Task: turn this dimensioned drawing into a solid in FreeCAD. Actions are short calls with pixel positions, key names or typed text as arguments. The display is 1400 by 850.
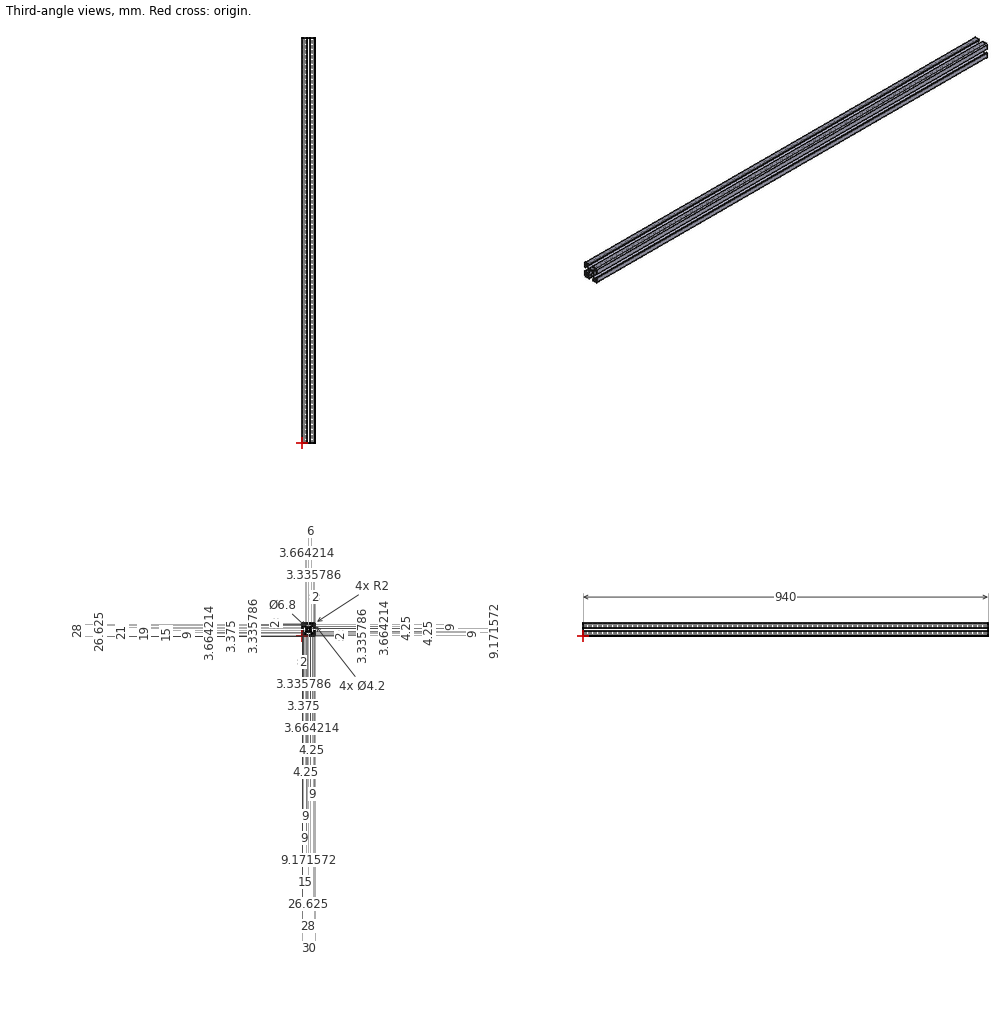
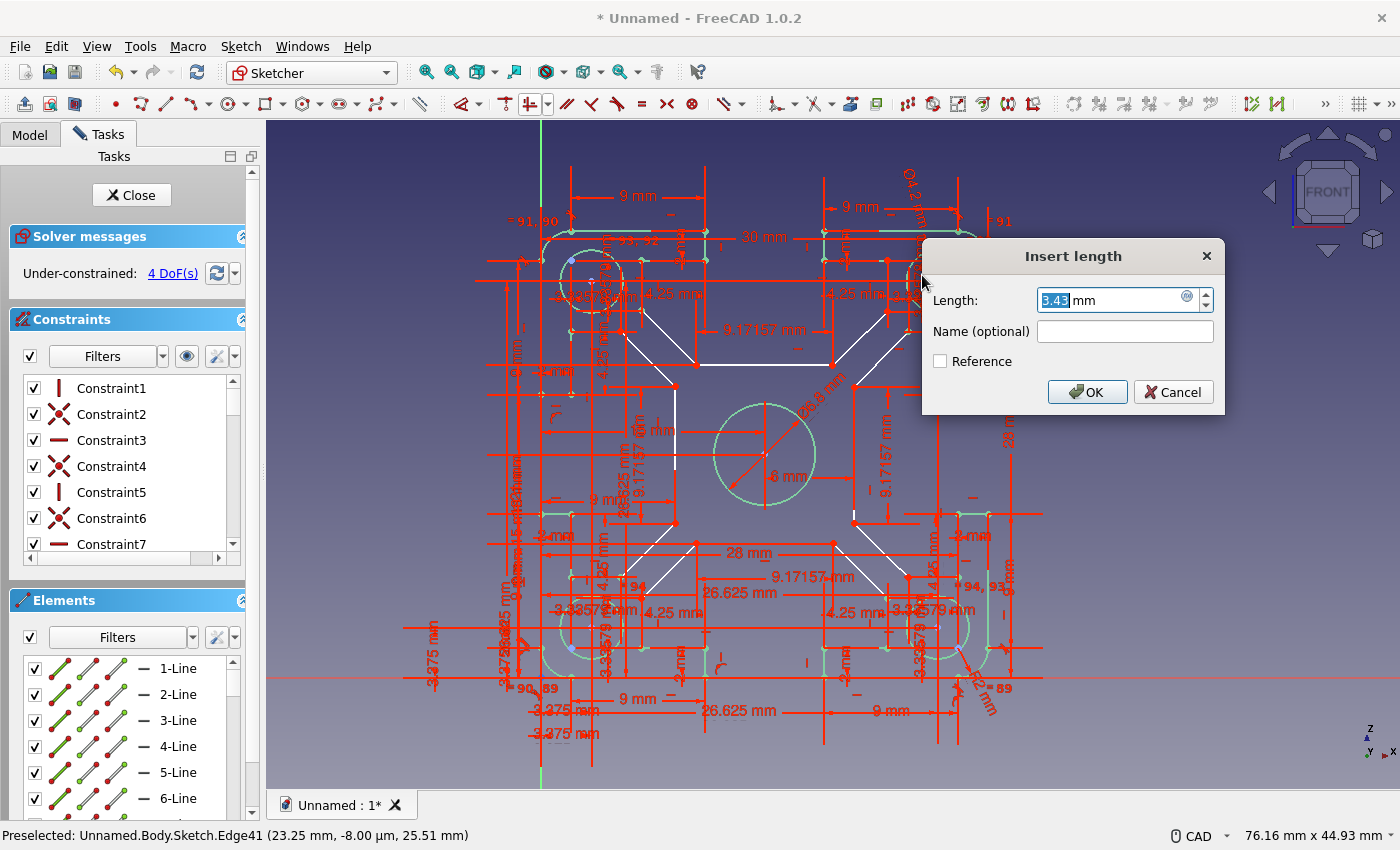
text(3.335786)
key(Return)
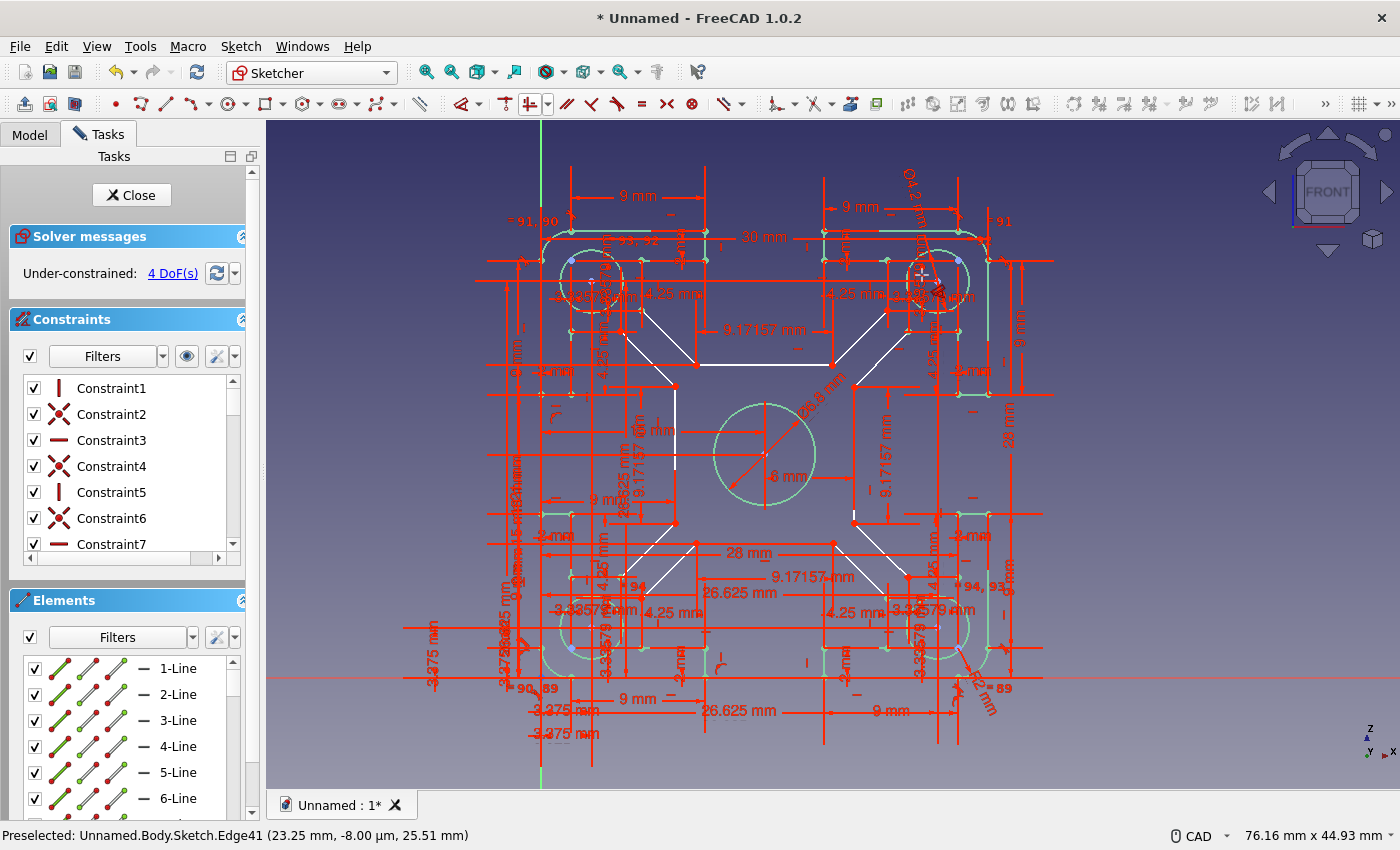
click(892, 348)
click(748, 379)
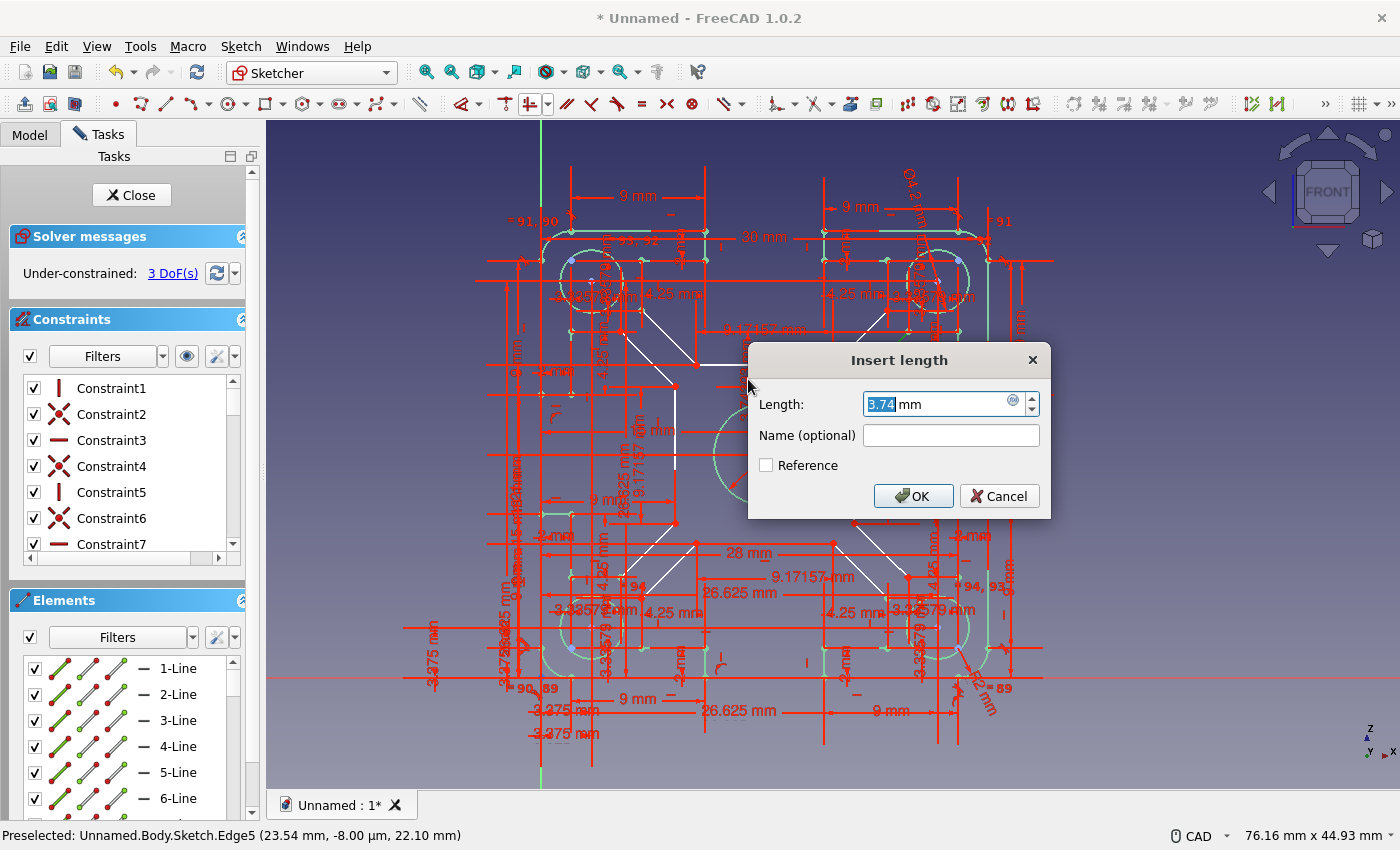
text(3.664214)
key(Return)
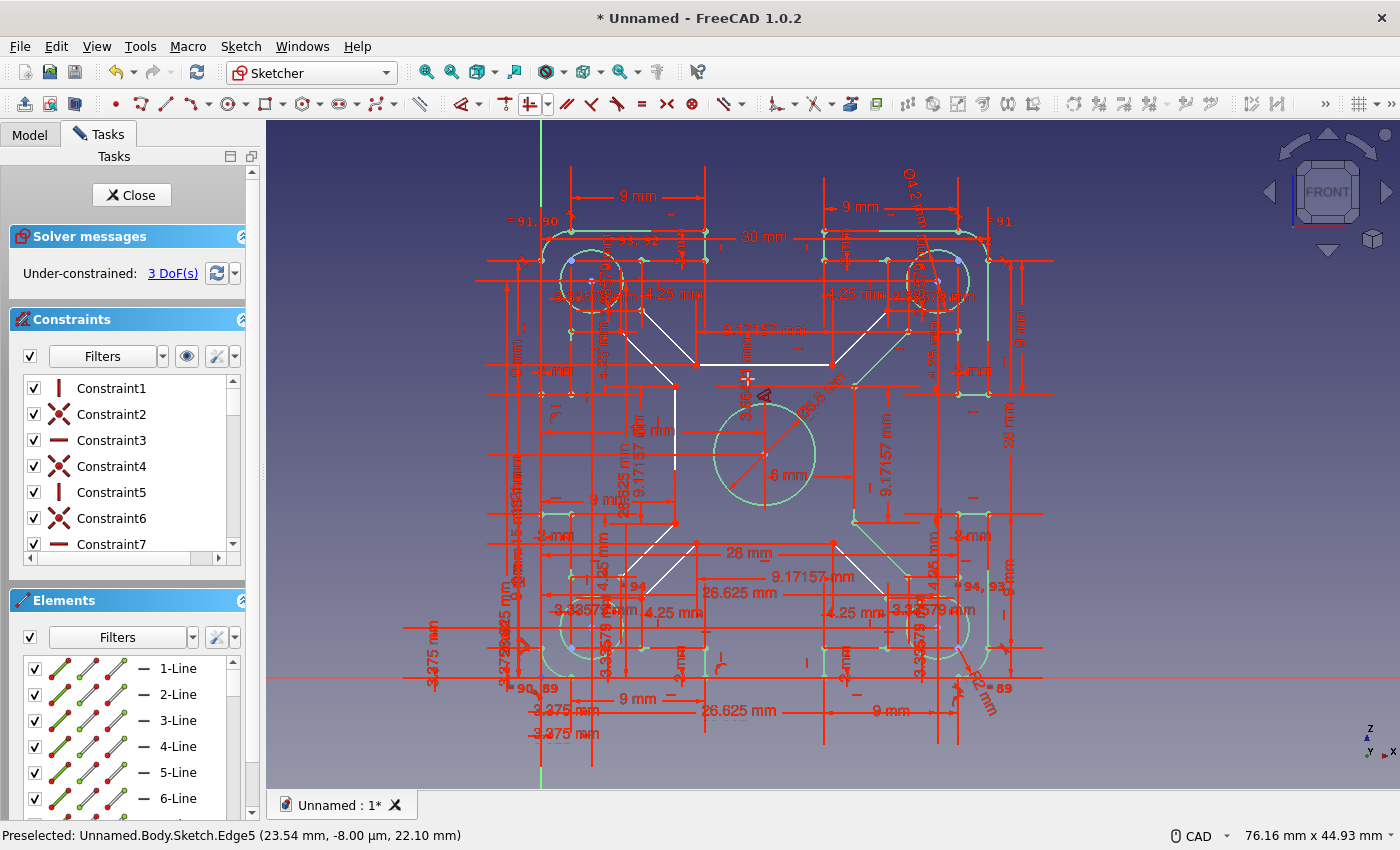
click(871, 582)
click(873, 510)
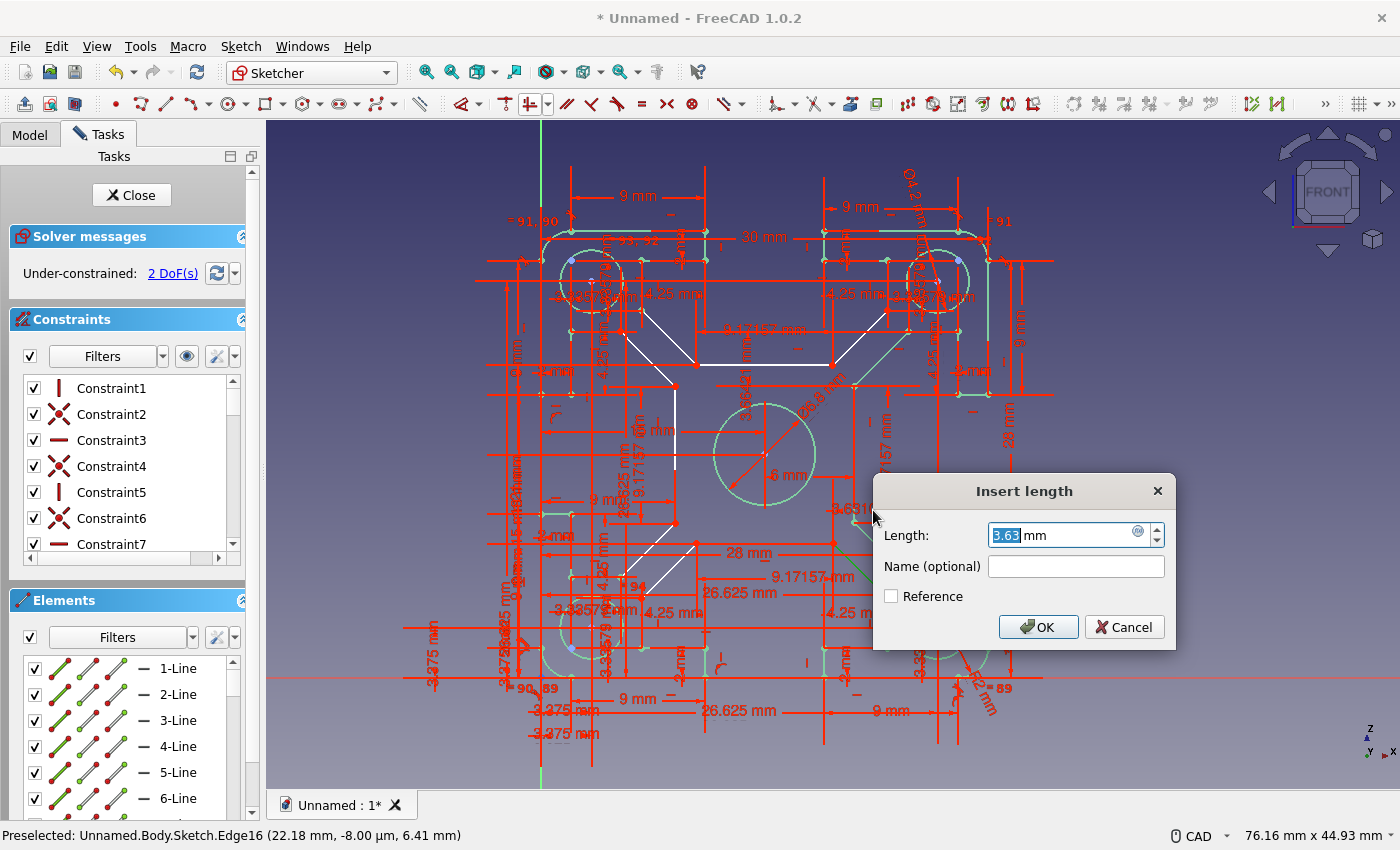
text(3.664214)
key(Return)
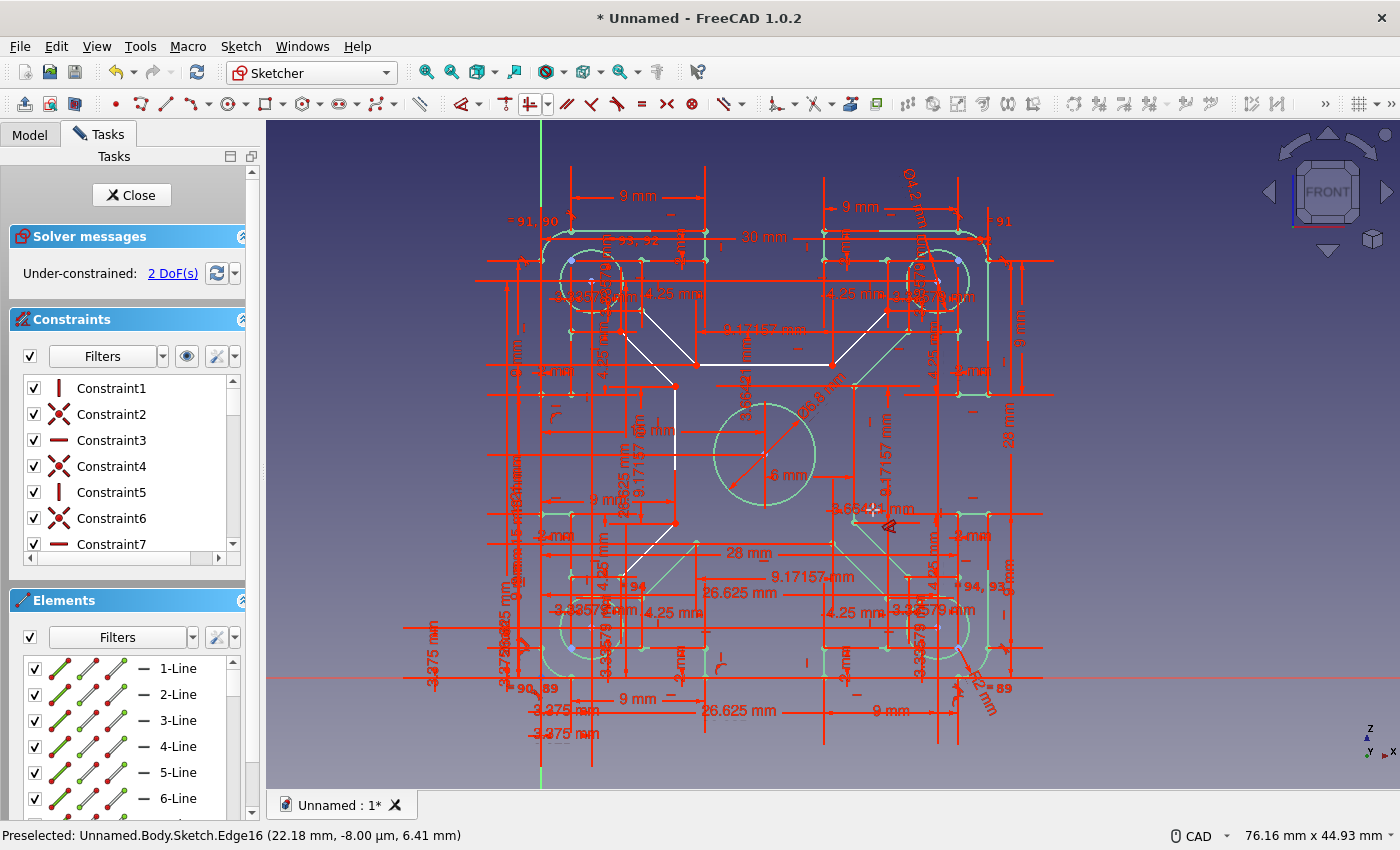
click(637, 561)
click(441, 550)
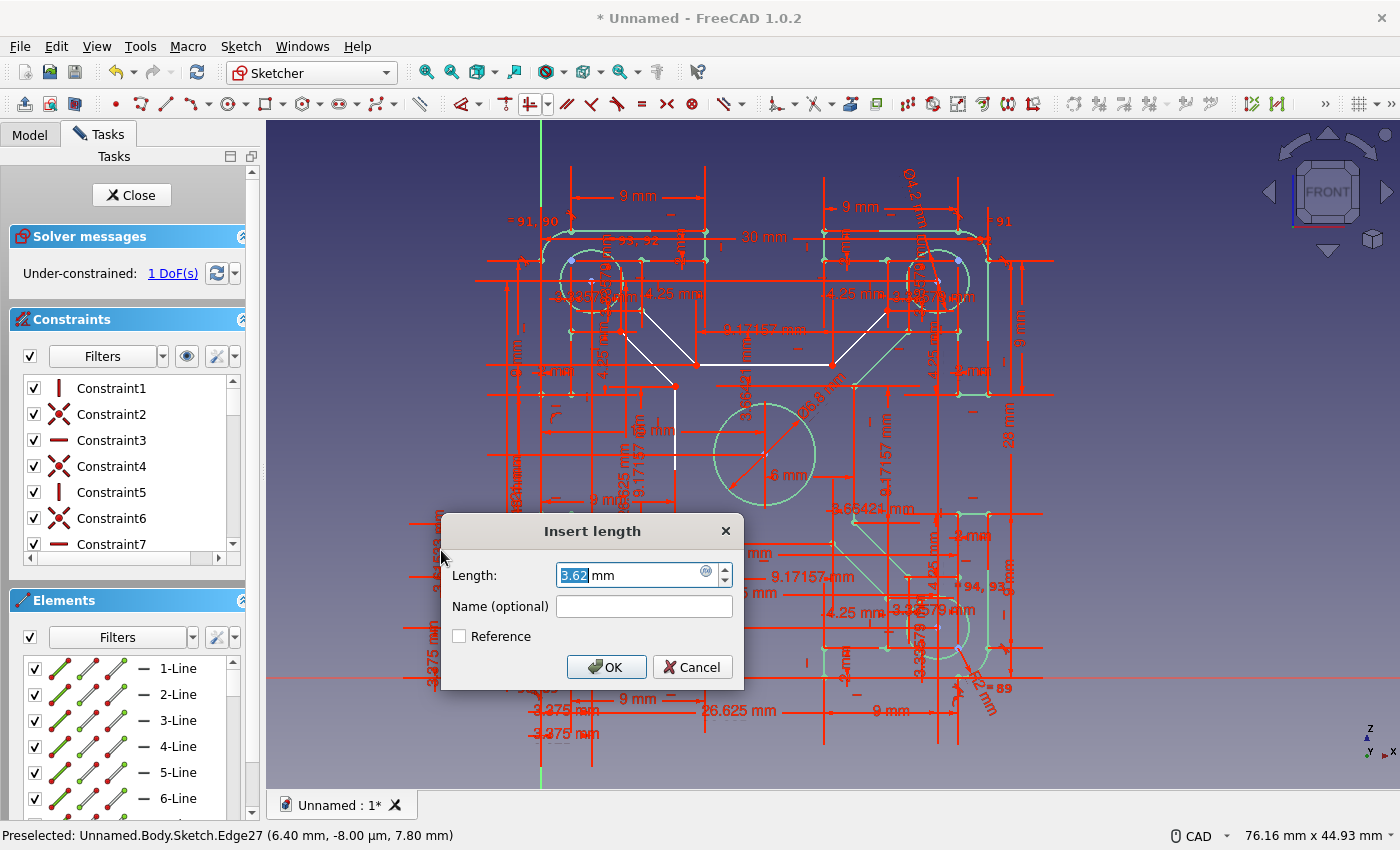
text(3.664214)
key(Return)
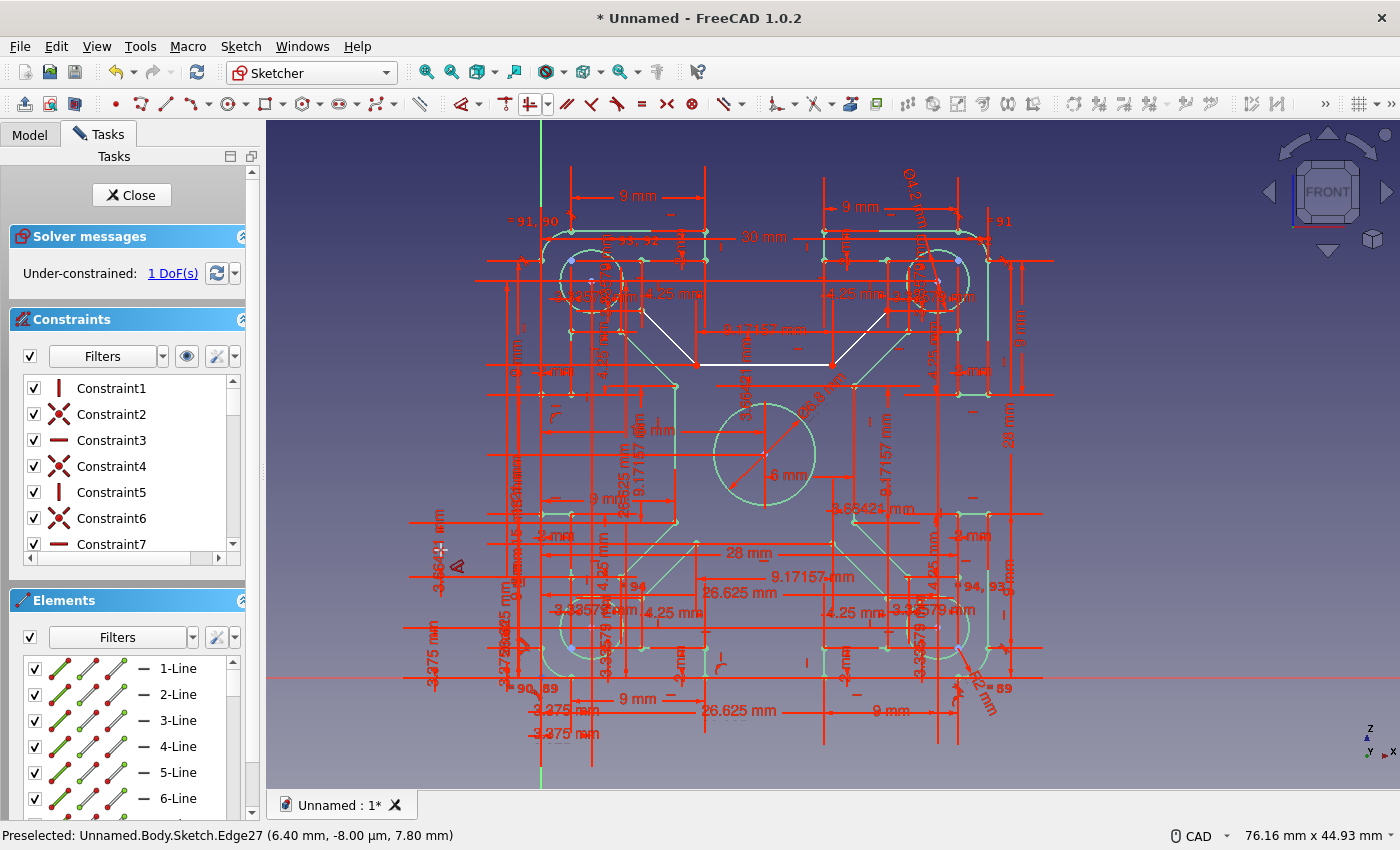
click(658, 327)
click(657, 399)